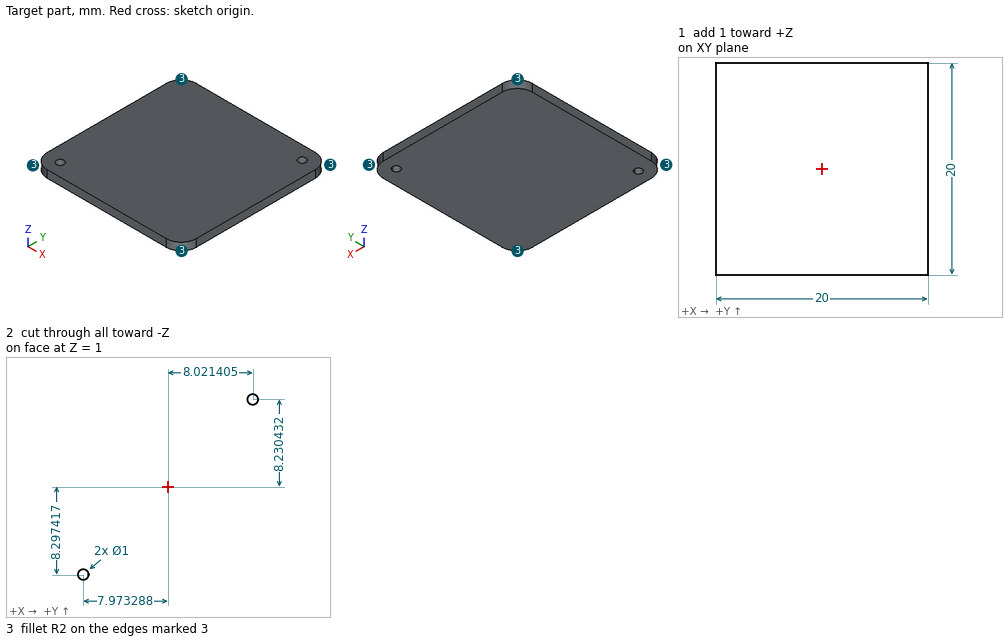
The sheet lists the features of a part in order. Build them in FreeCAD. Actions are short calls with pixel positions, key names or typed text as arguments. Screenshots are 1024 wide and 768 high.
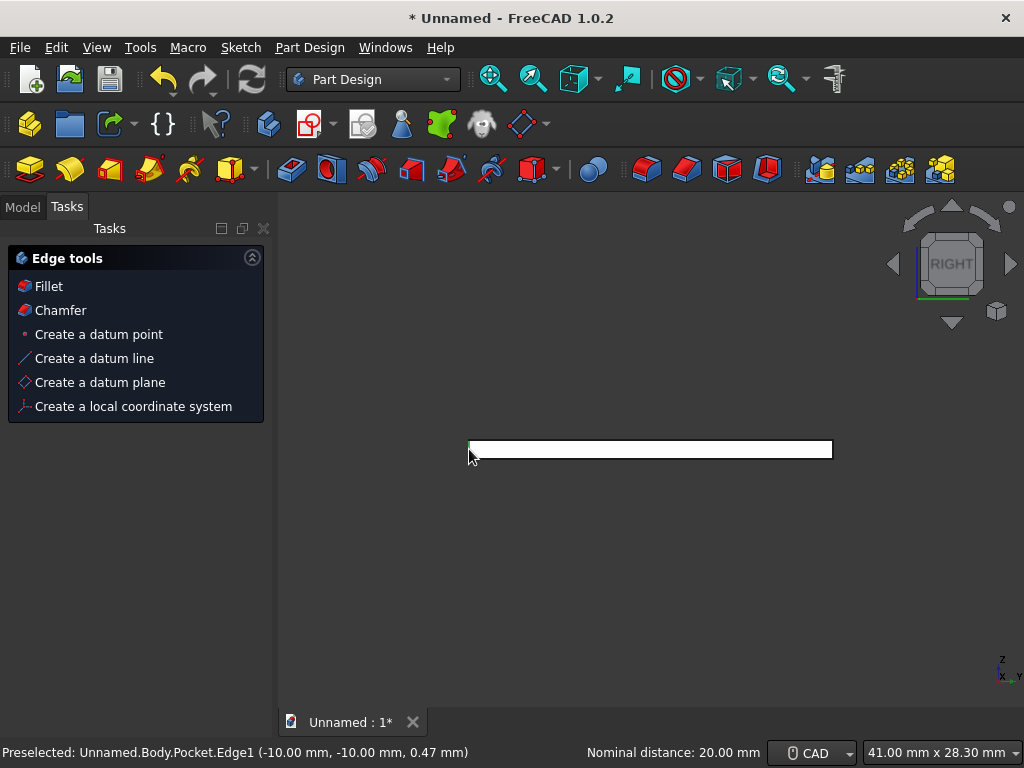
click(833, 448, ctrl)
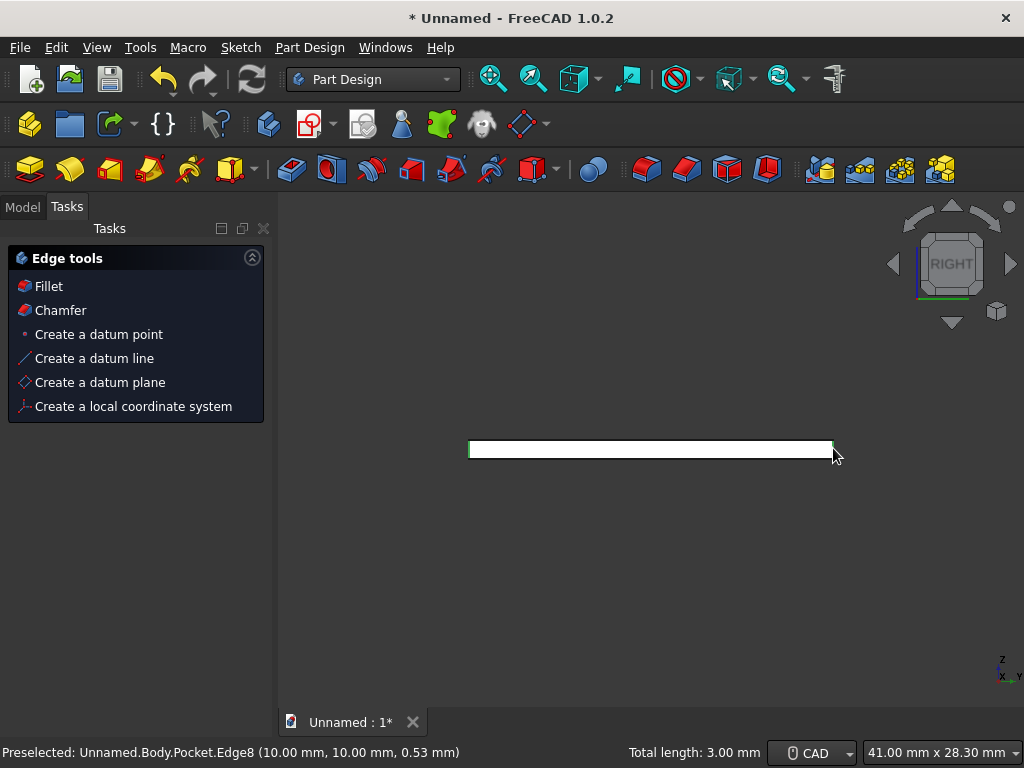
scroll(833, 448, up, 4)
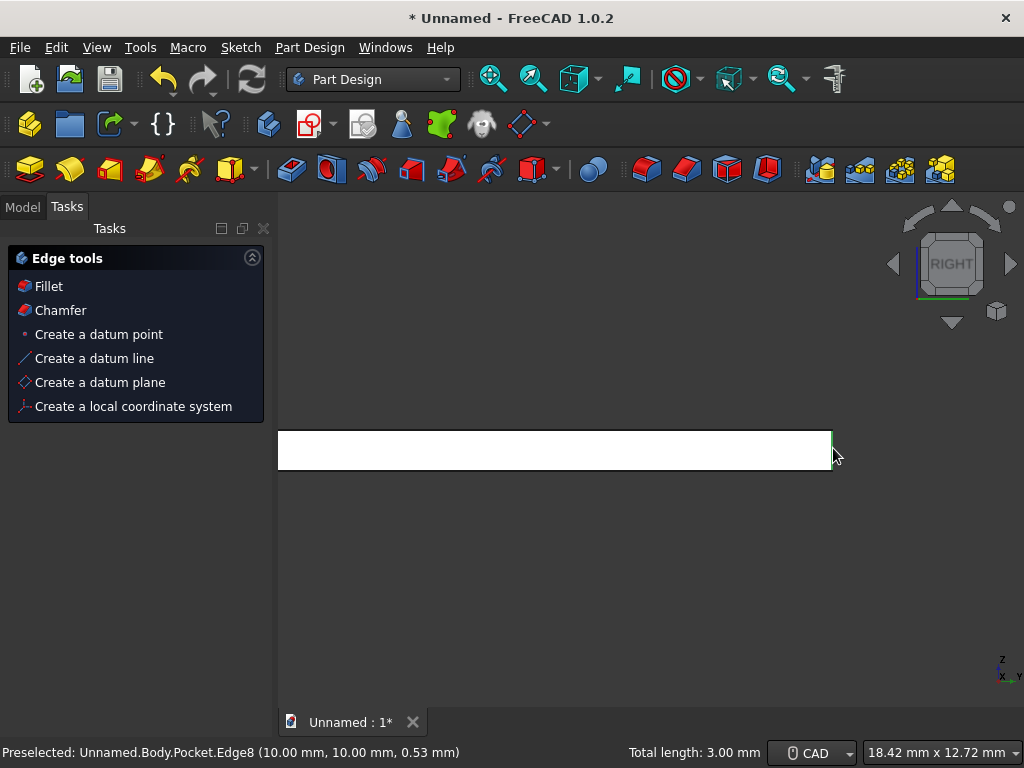
key(v)
key(f)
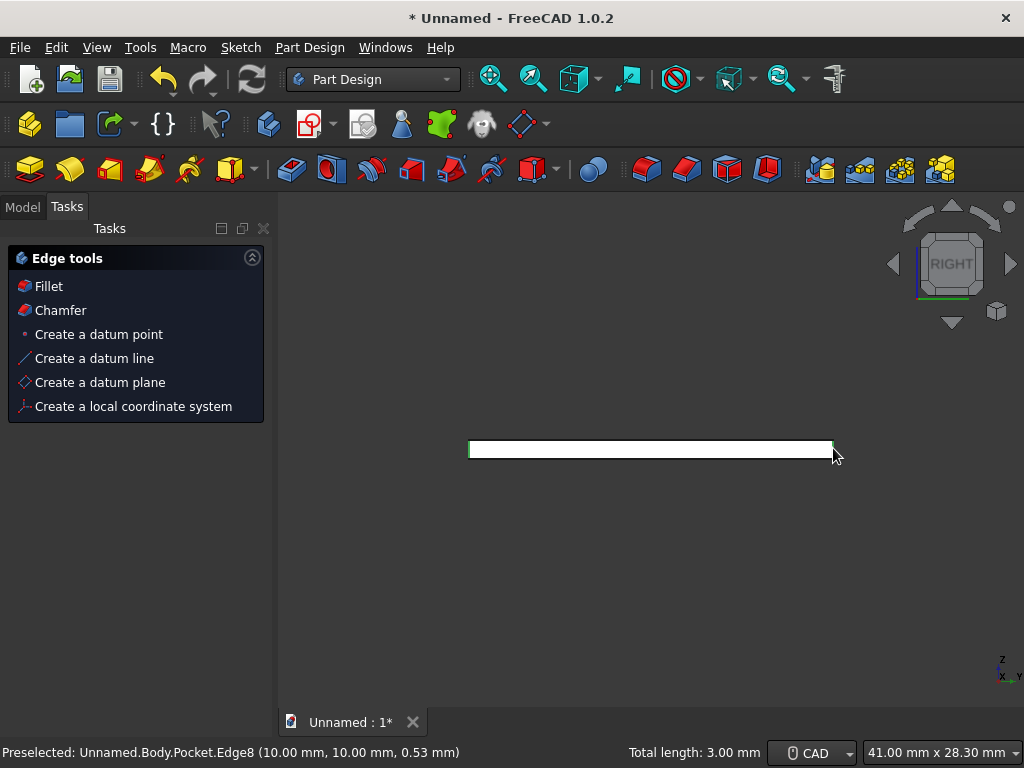
key(5)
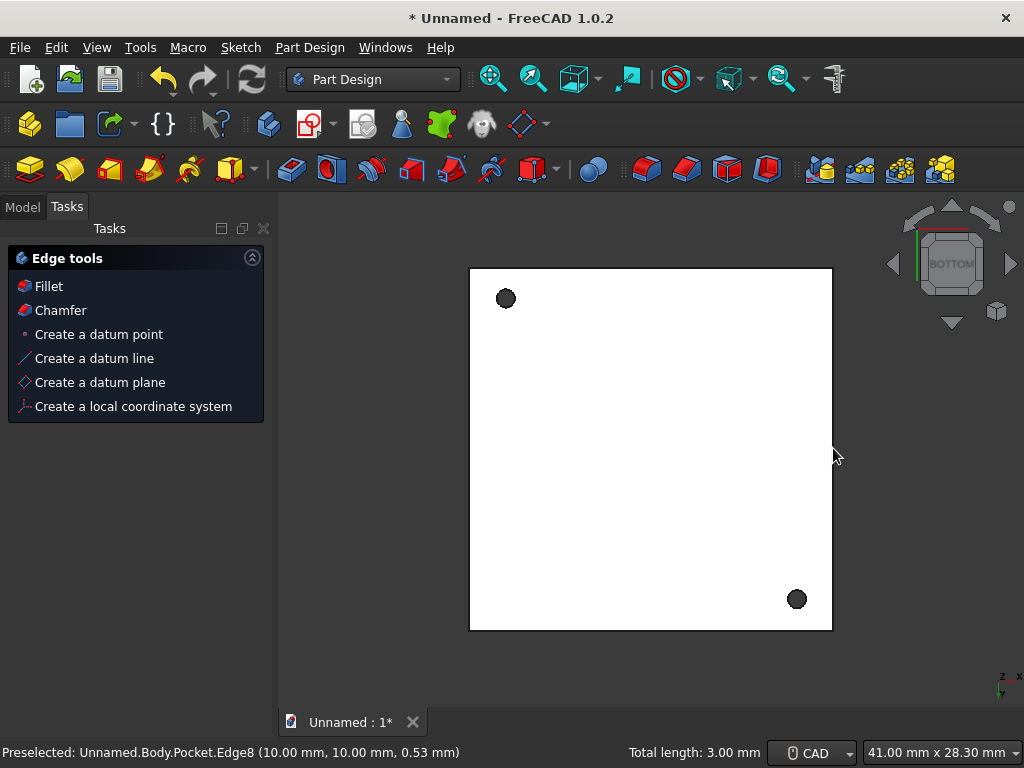
scroll(469, 630, up, 4)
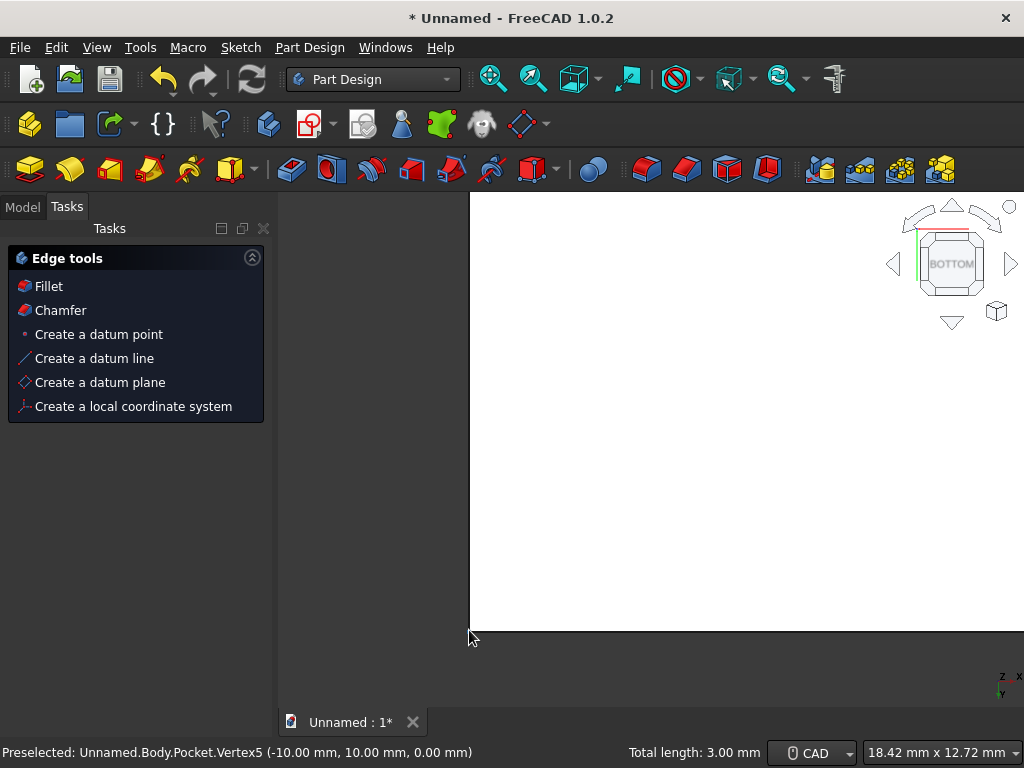
click(494, 80)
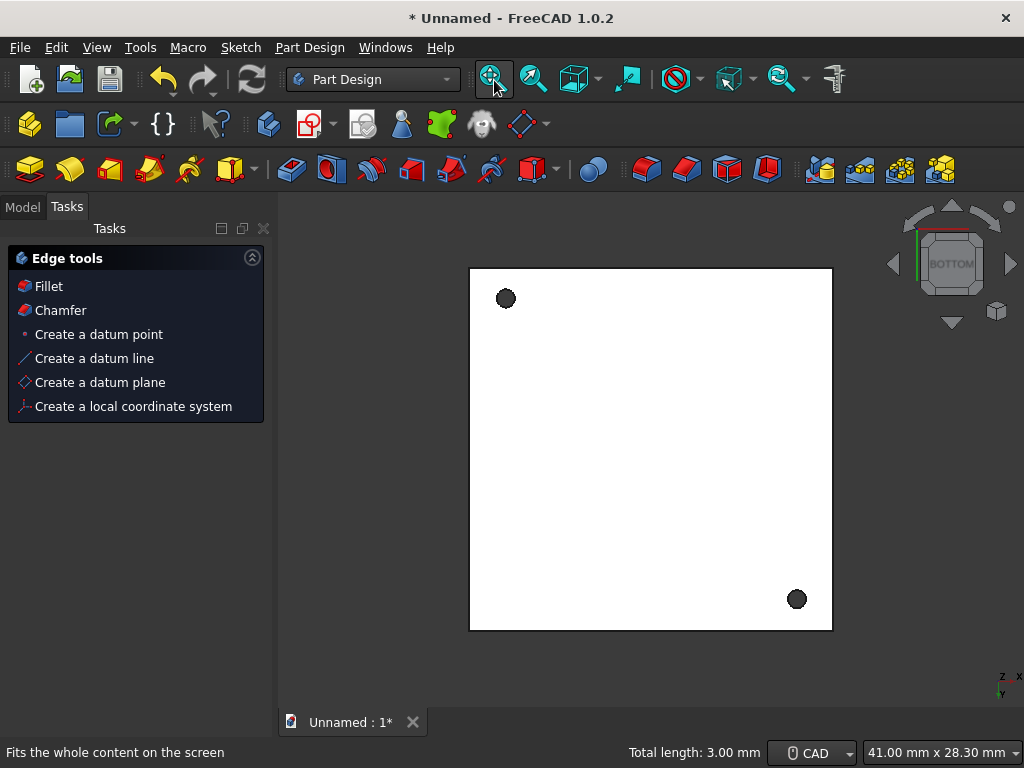
key(4)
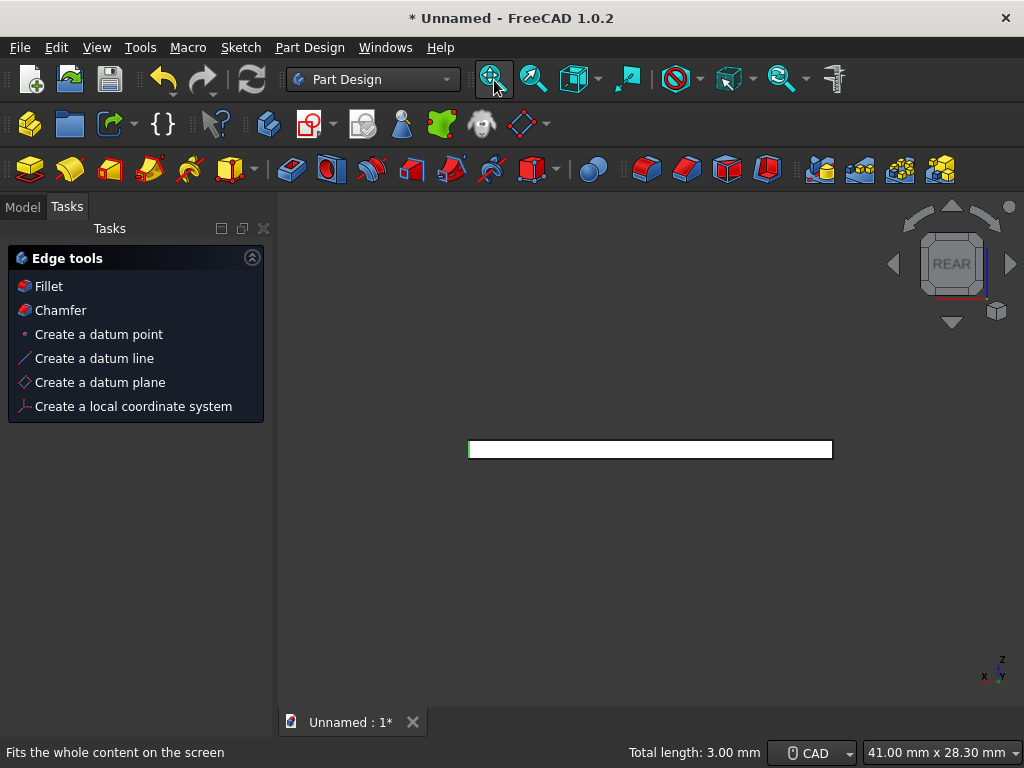
click(833, 449, ctrl)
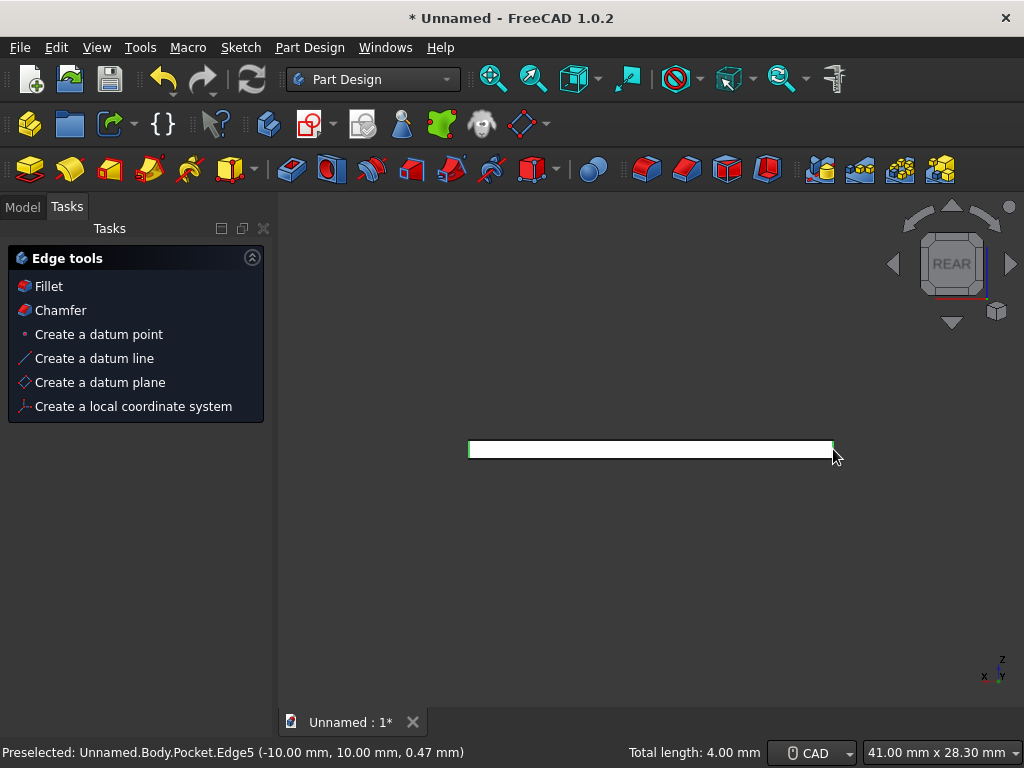
click(648, 170)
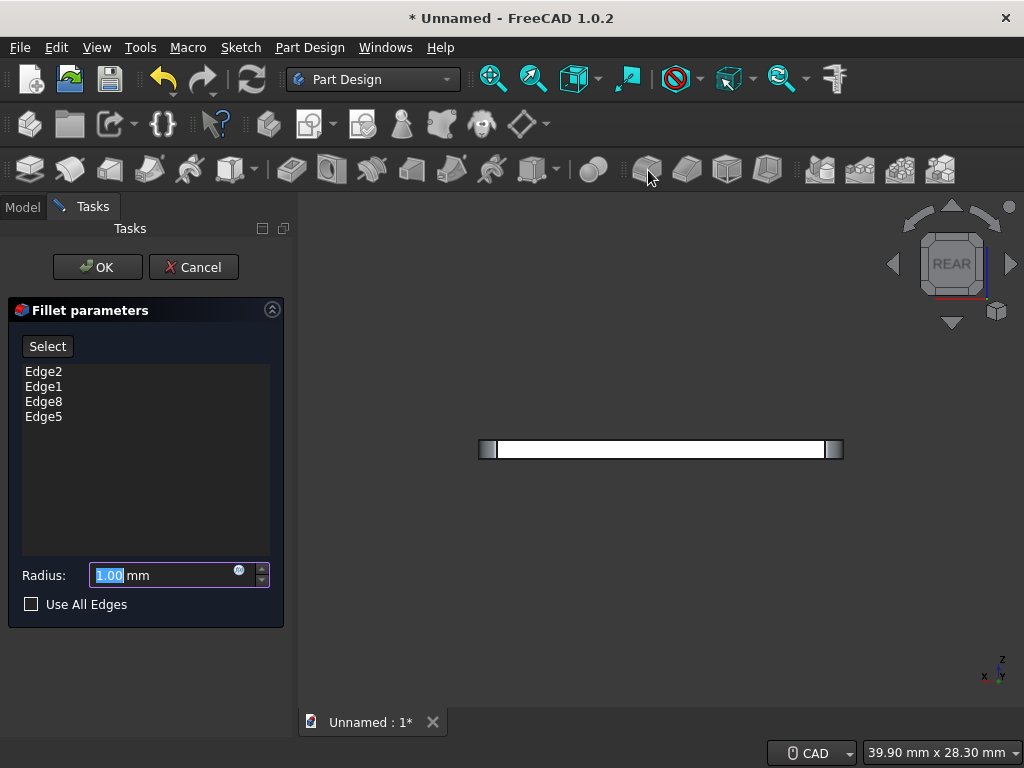
text(2)
key(Tab)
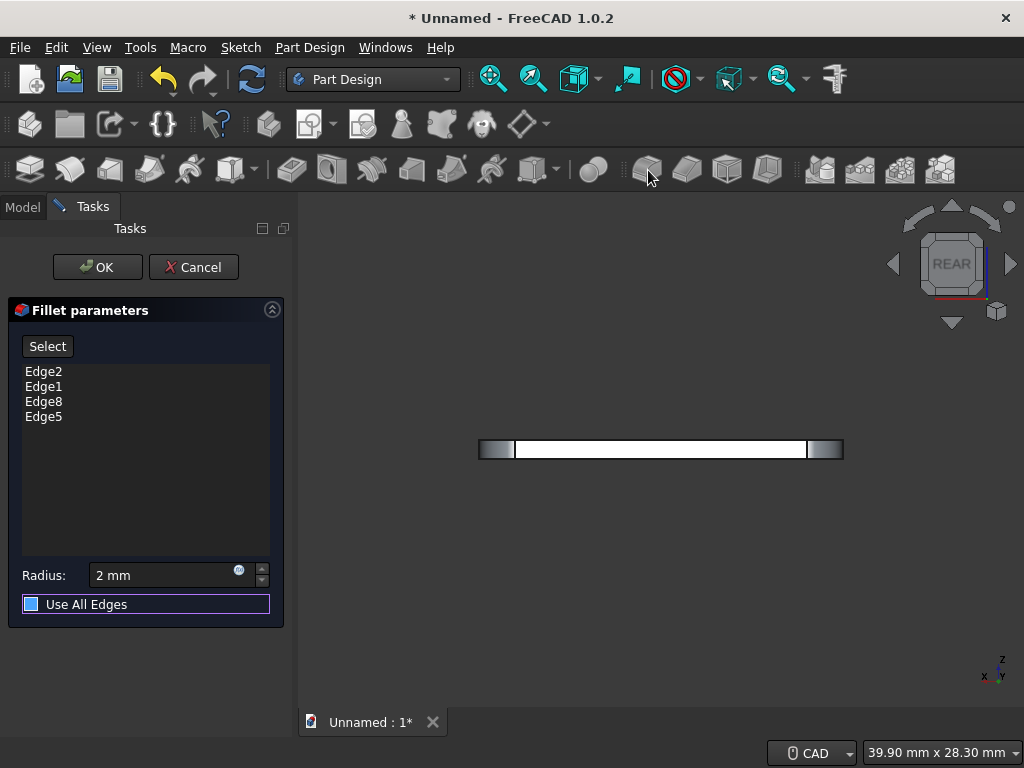
click(98, 267)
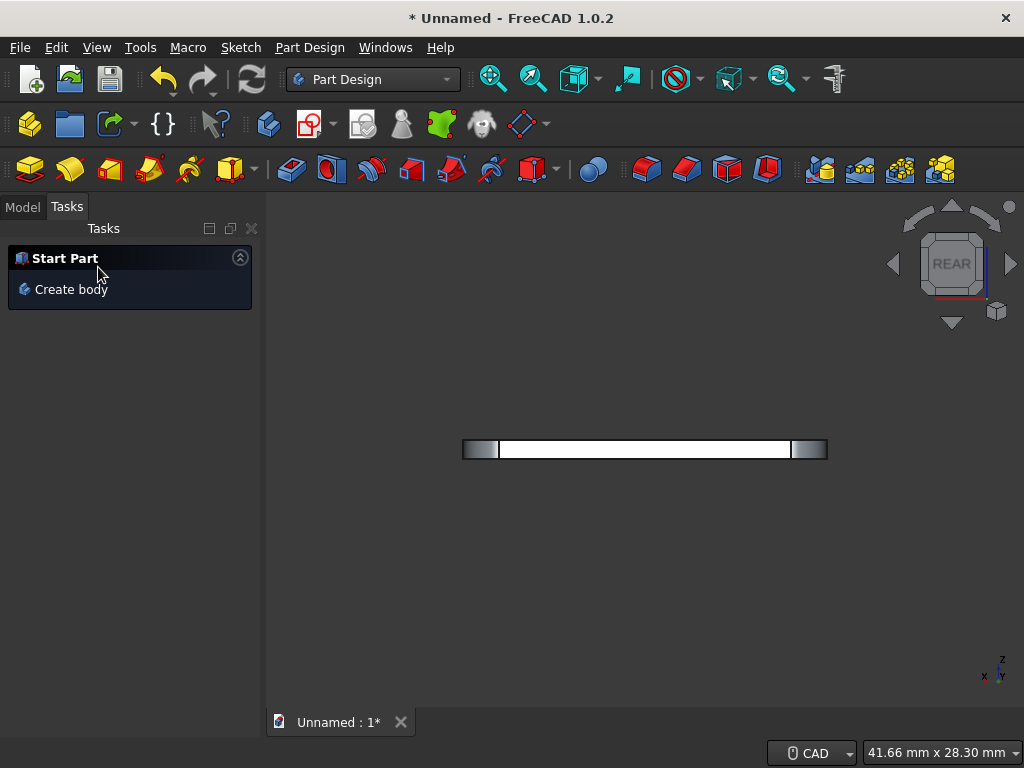
key(0)